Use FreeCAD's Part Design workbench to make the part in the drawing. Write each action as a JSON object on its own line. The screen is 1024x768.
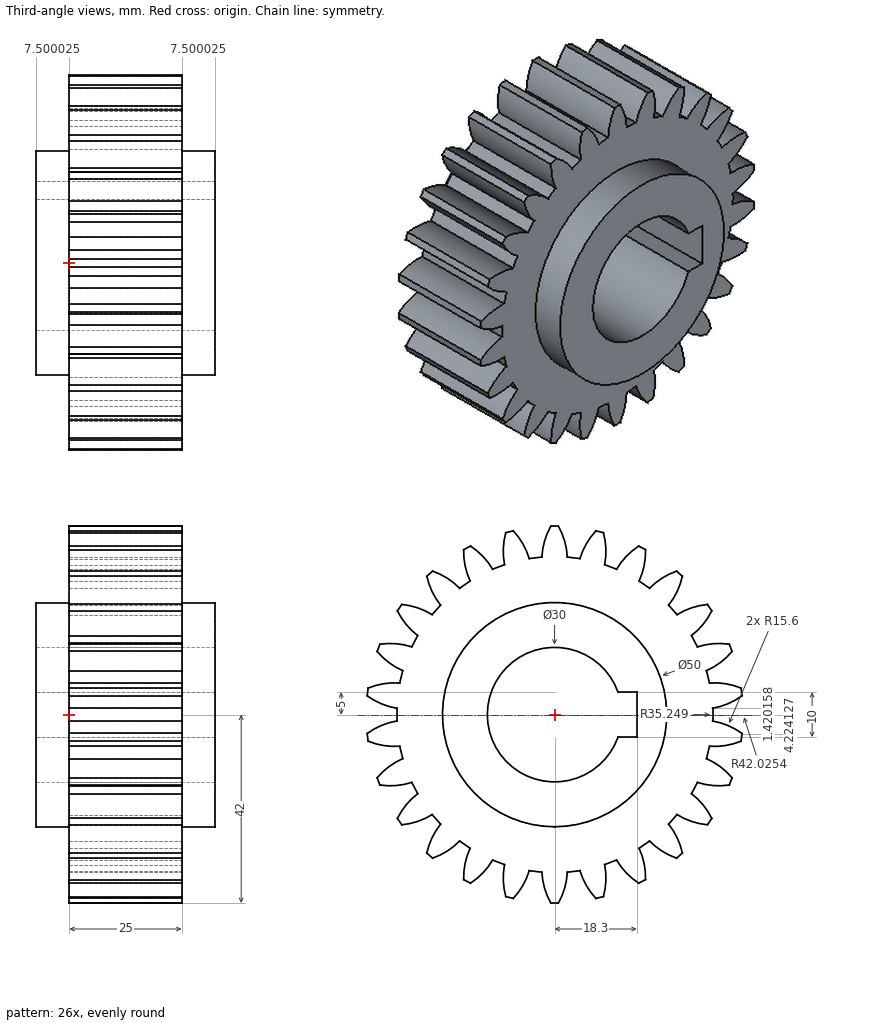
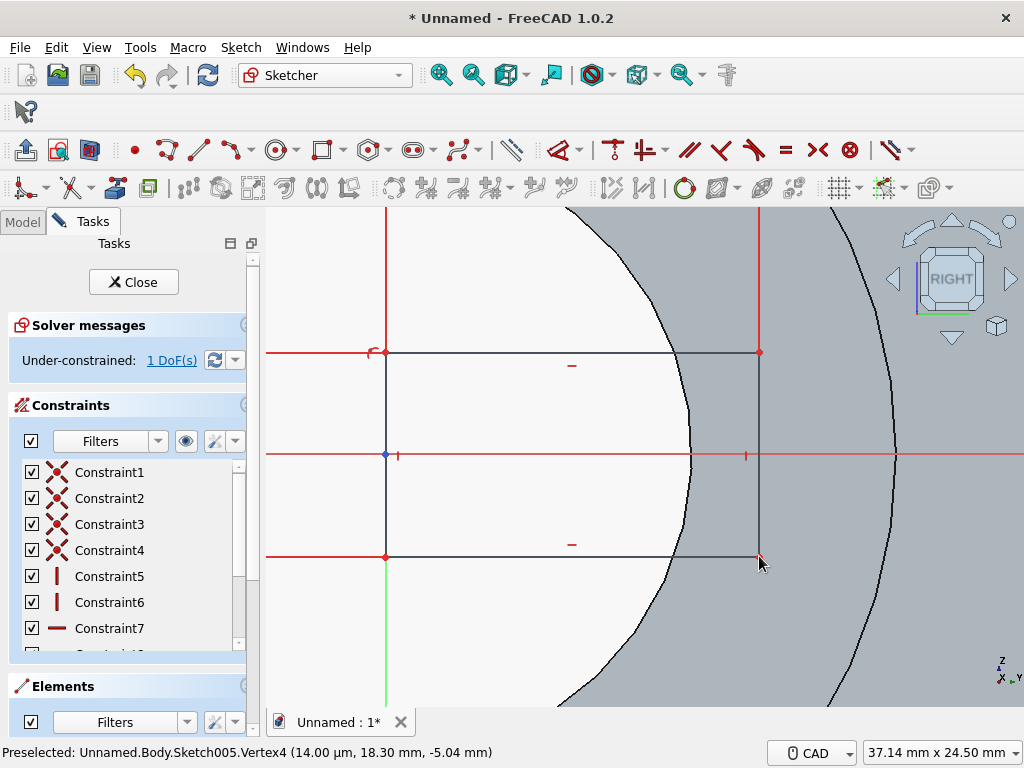
{"action": "left_click", "coordinate": [558, 150]}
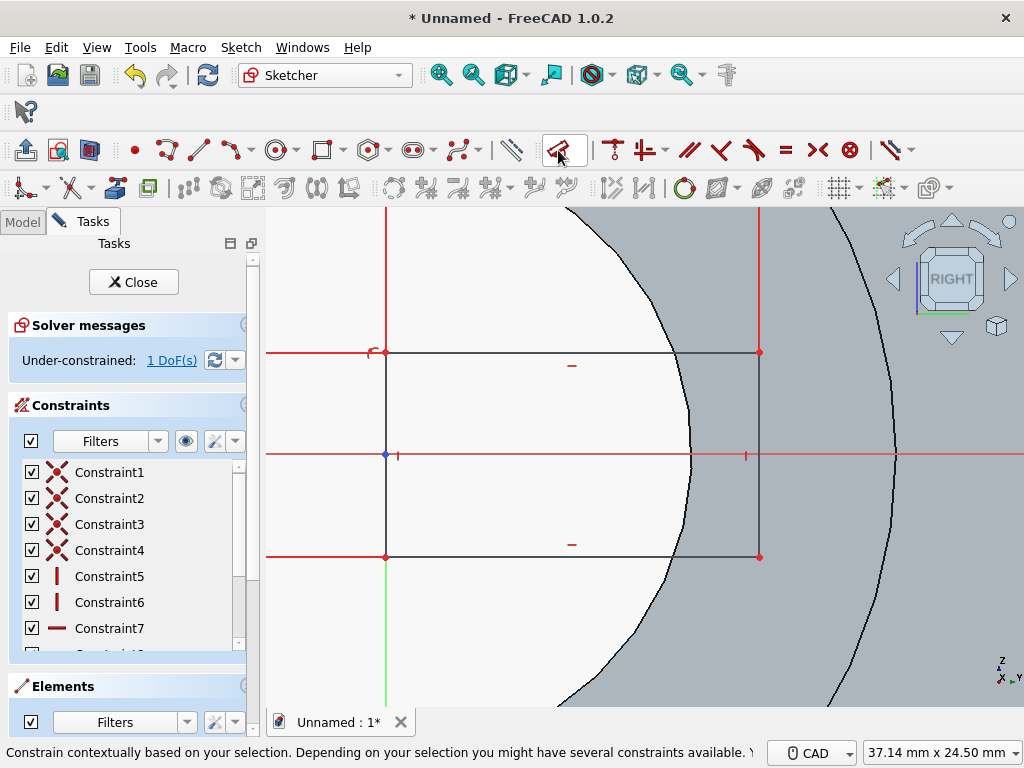
{"action": "left_click", "coordinate": [386, 353]}
{"action": "left_click", "coordinate": [352, 404]}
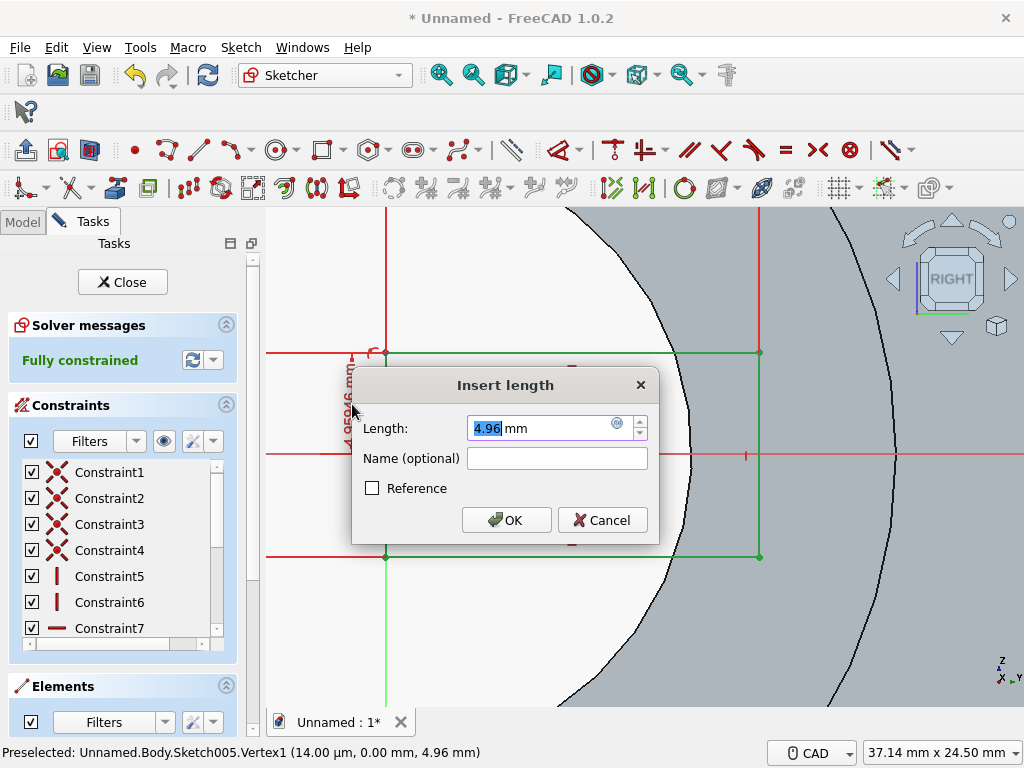
{"action": "type", "text": "5"}
{"action": "key", "text": "Return"}
{"action": "key", "text": "Escape"}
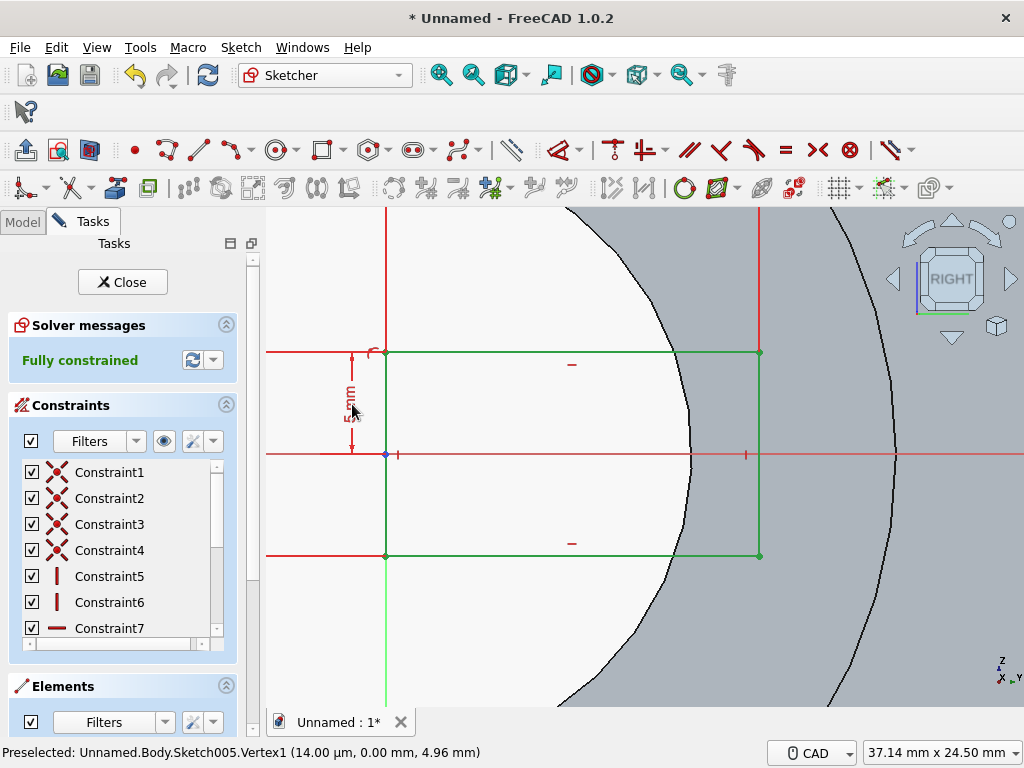
{"action": "left_click", "coordinate": [123, 282]}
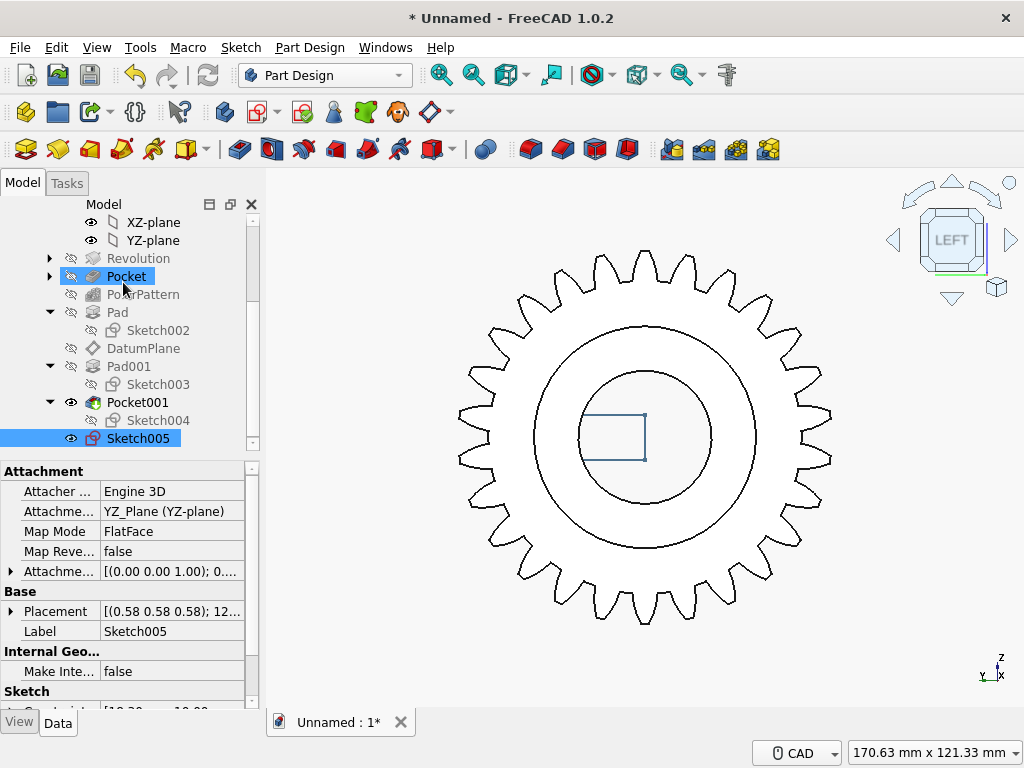
{"action": "left_click", "coordinate": [240, 150]}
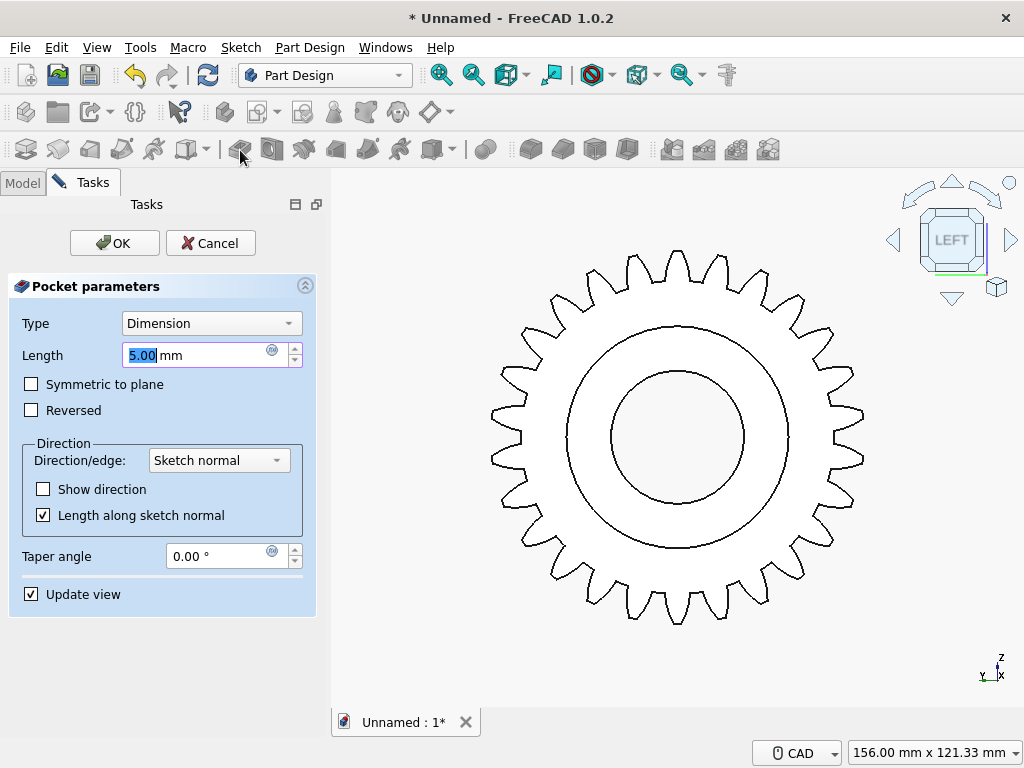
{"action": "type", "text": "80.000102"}
{"action": "key", "text": "Tab"}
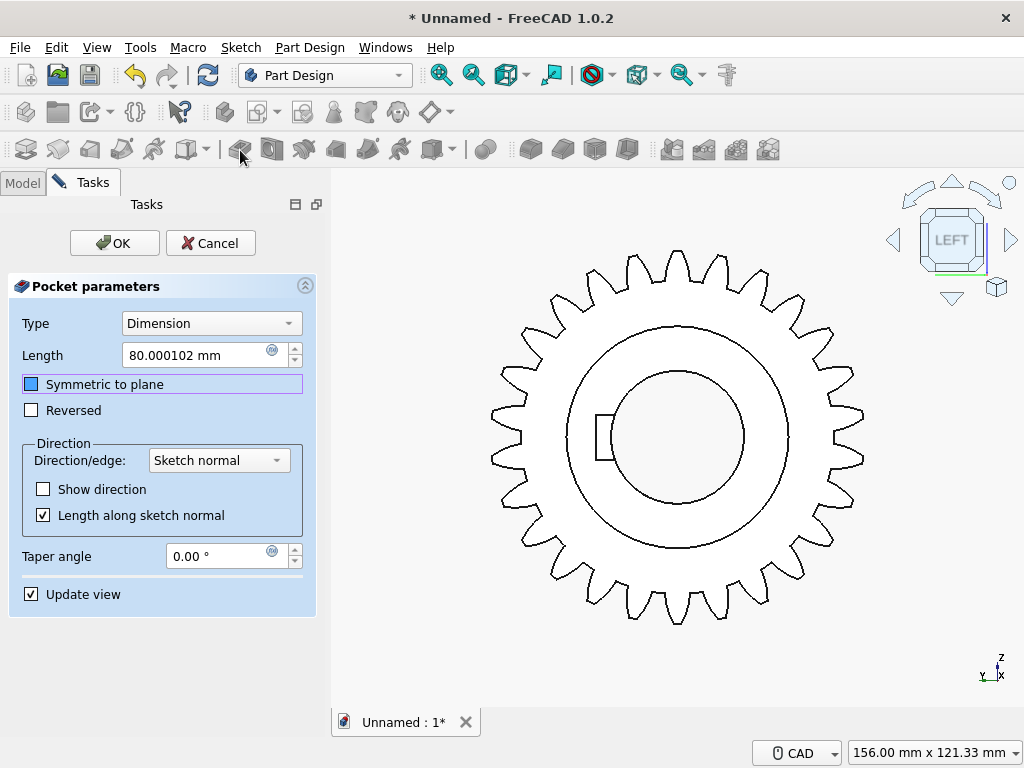
{"action": "left_click", "coordinate": [30, 384]}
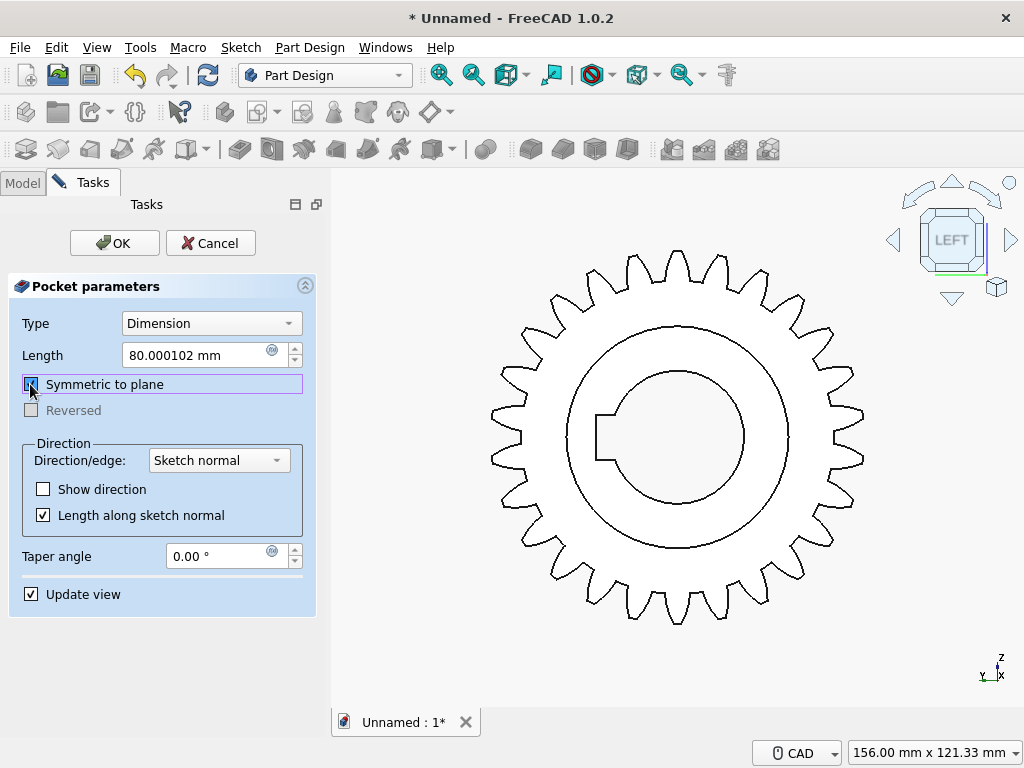
{"action": "left_click", "coordinate": [115, 243]}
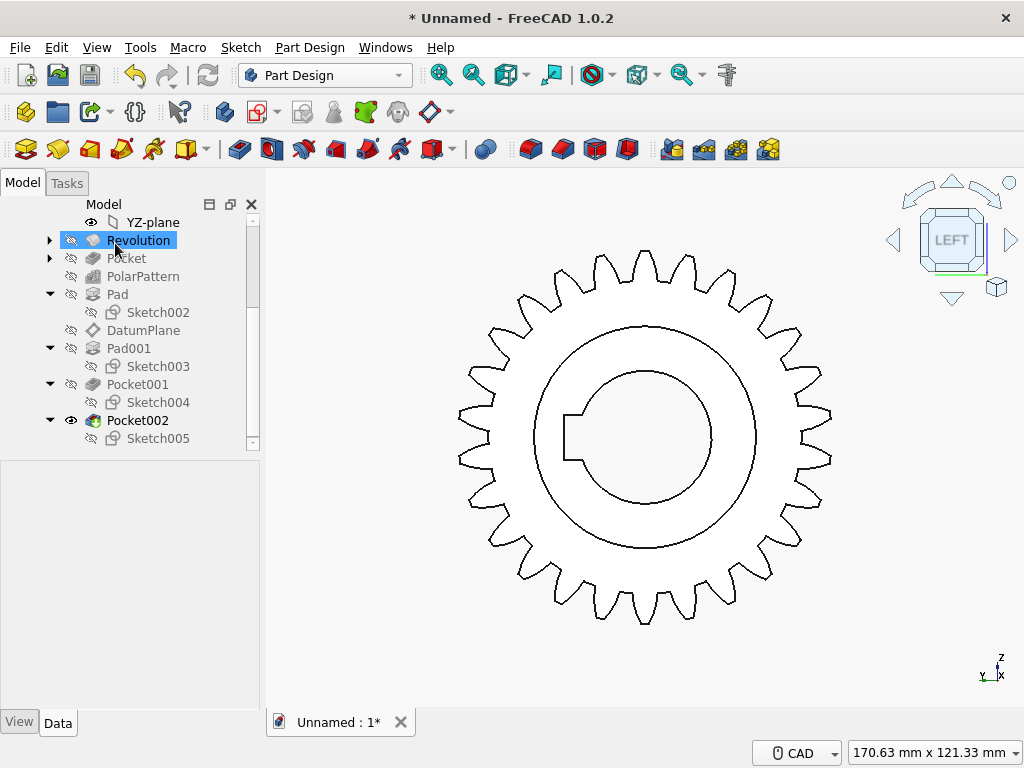
{"action": "key", "text": "0"}